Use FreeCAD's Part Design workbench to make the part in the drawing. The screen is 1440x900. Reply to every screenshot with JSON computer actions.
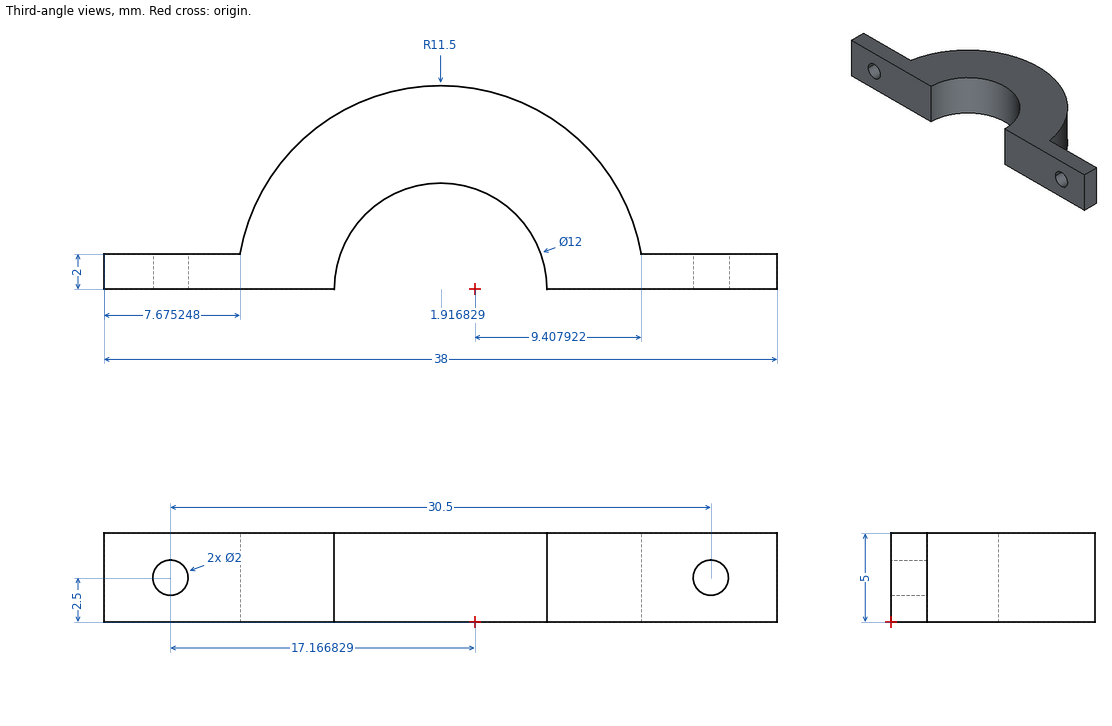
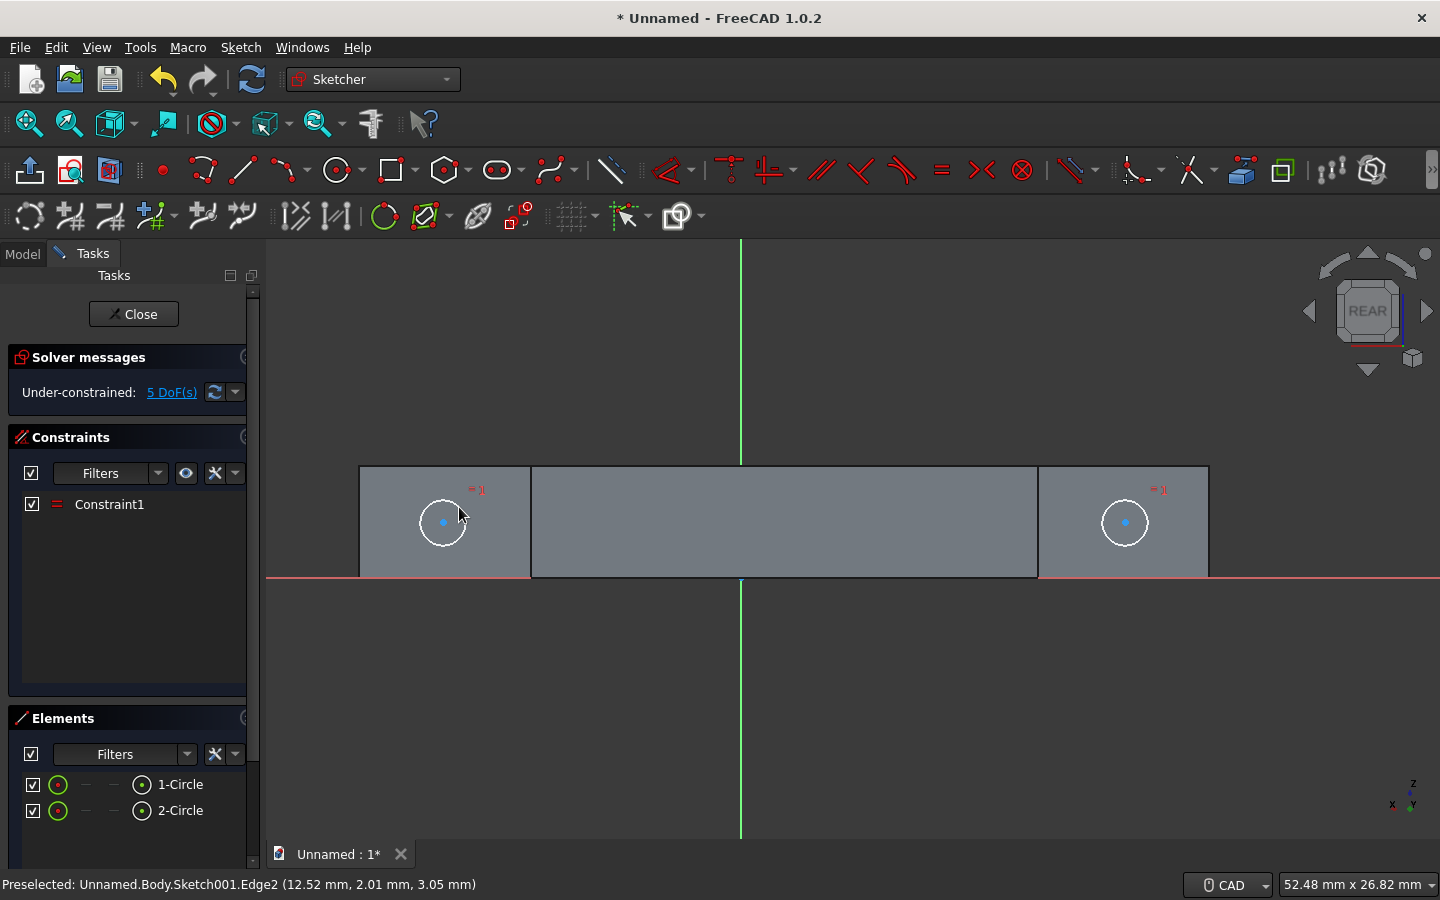
{"action": "left_click", "coordinate": [1125, 523]}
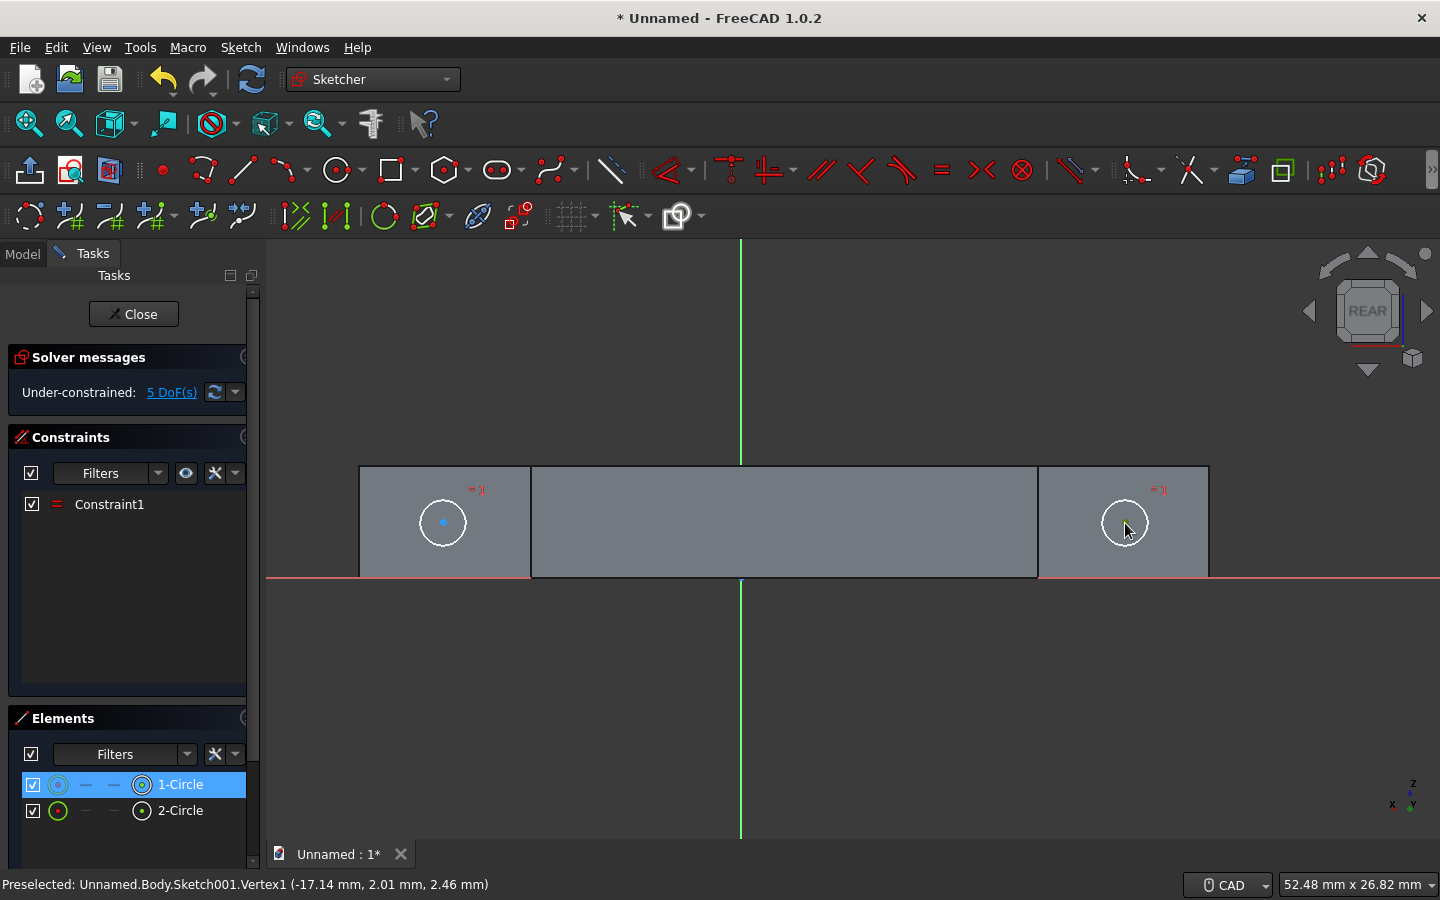
{"action": "left_click", "coordinate": [443, 523]}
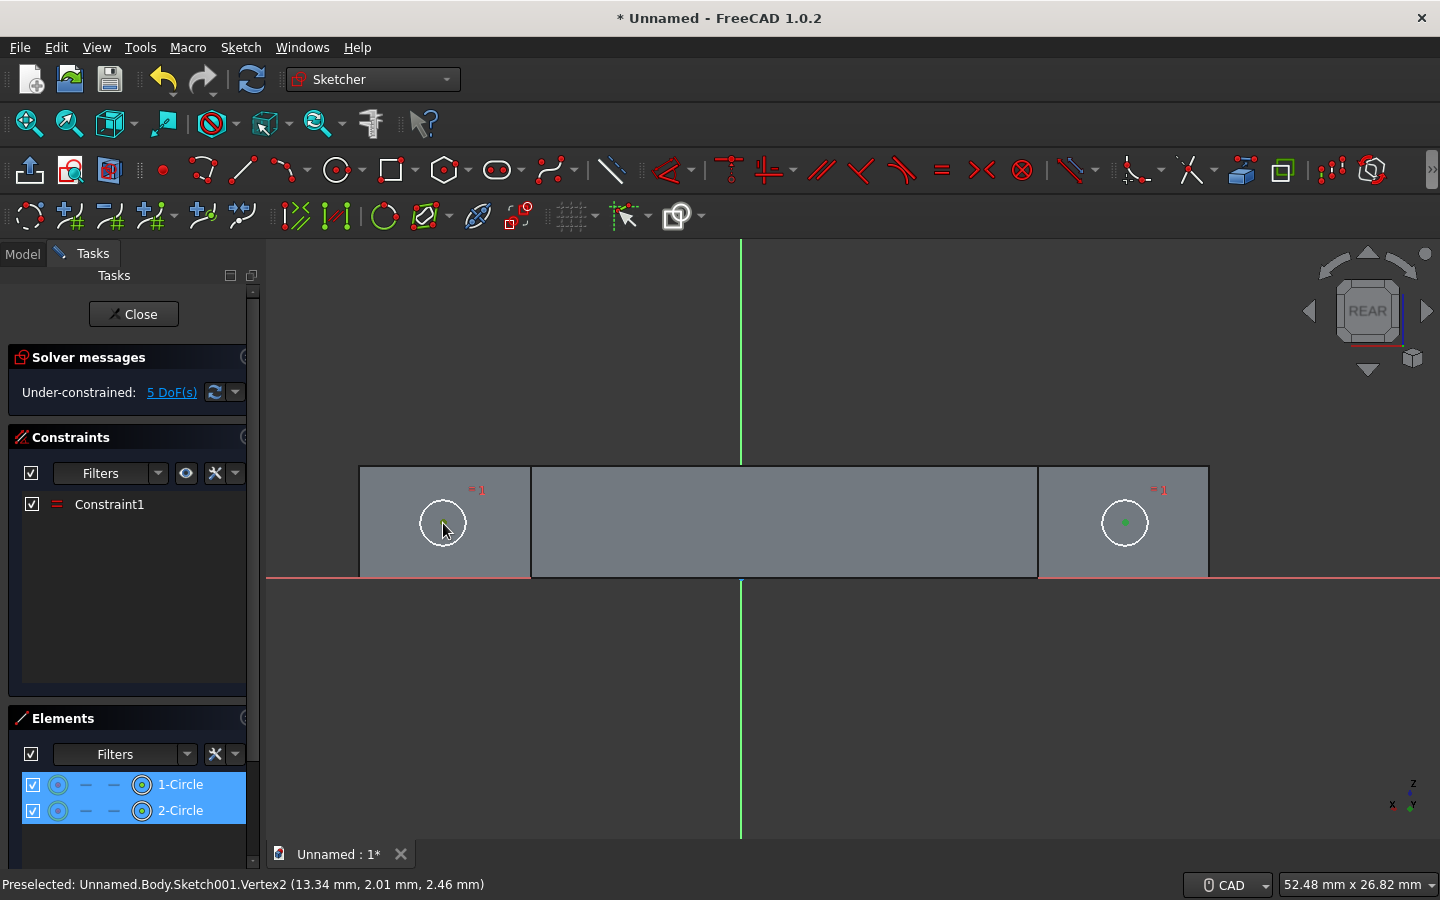
{"action": "key", "text": "h"}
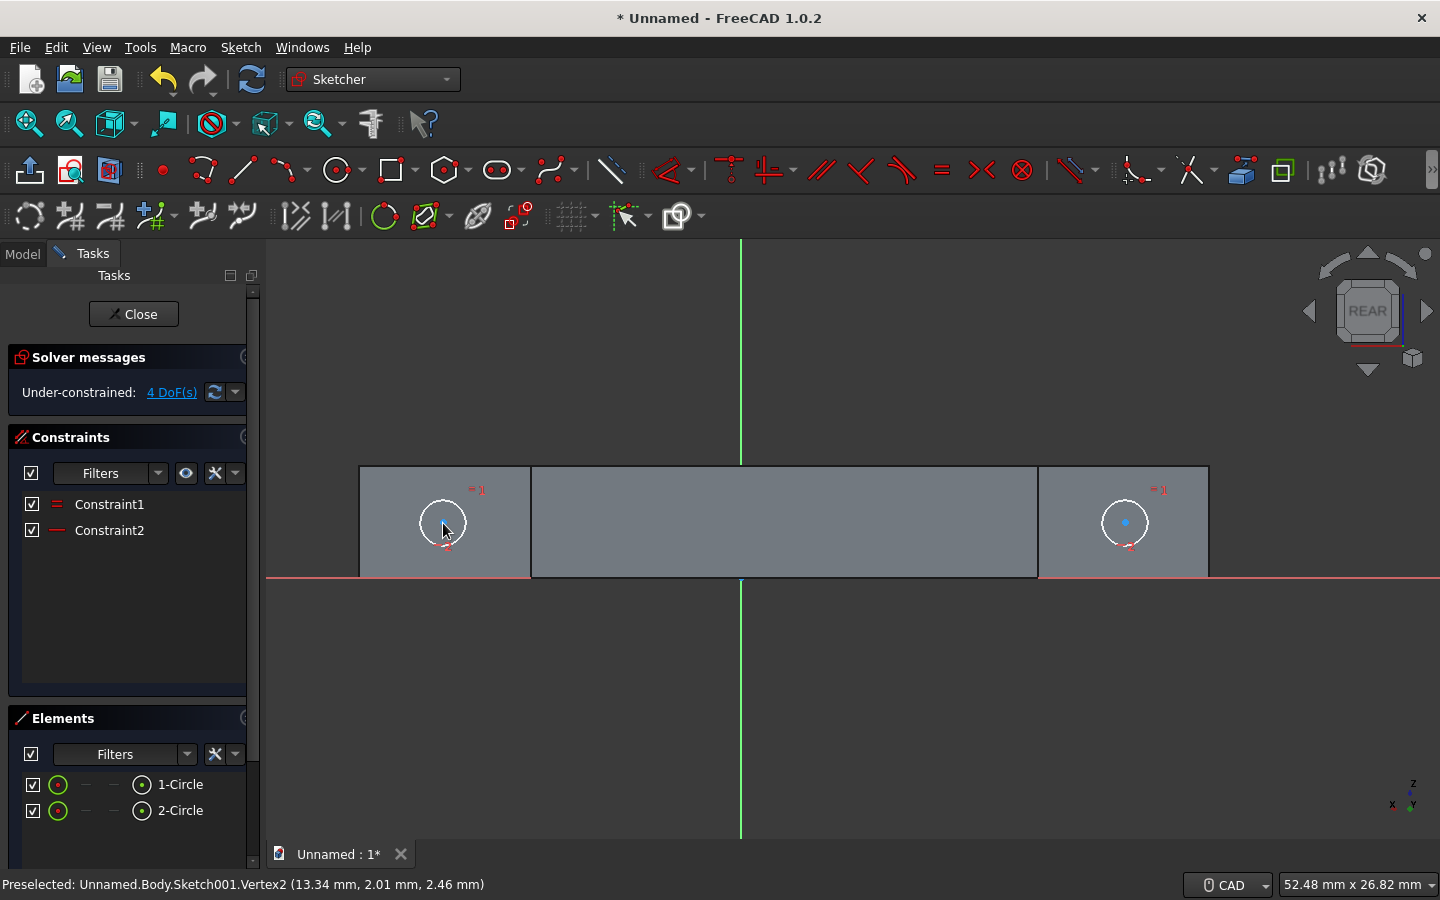
{"action": "left_click", "coordinate": [666, 170]}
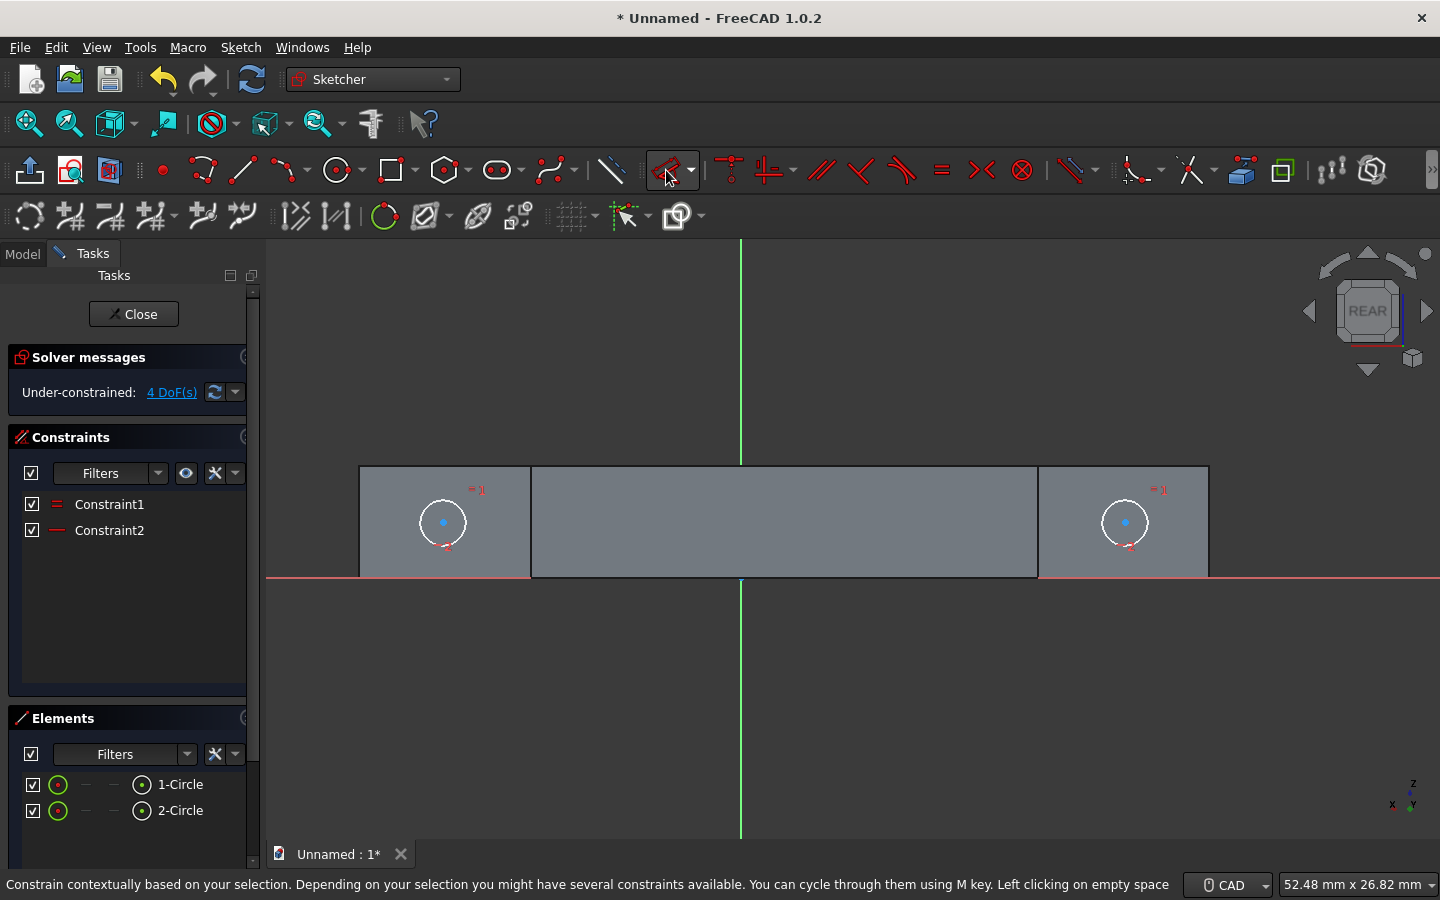
{"action": "left_click", "coordinate": [1141, 507]}
{"action": "left_click", "coordinate": [1164, 484]}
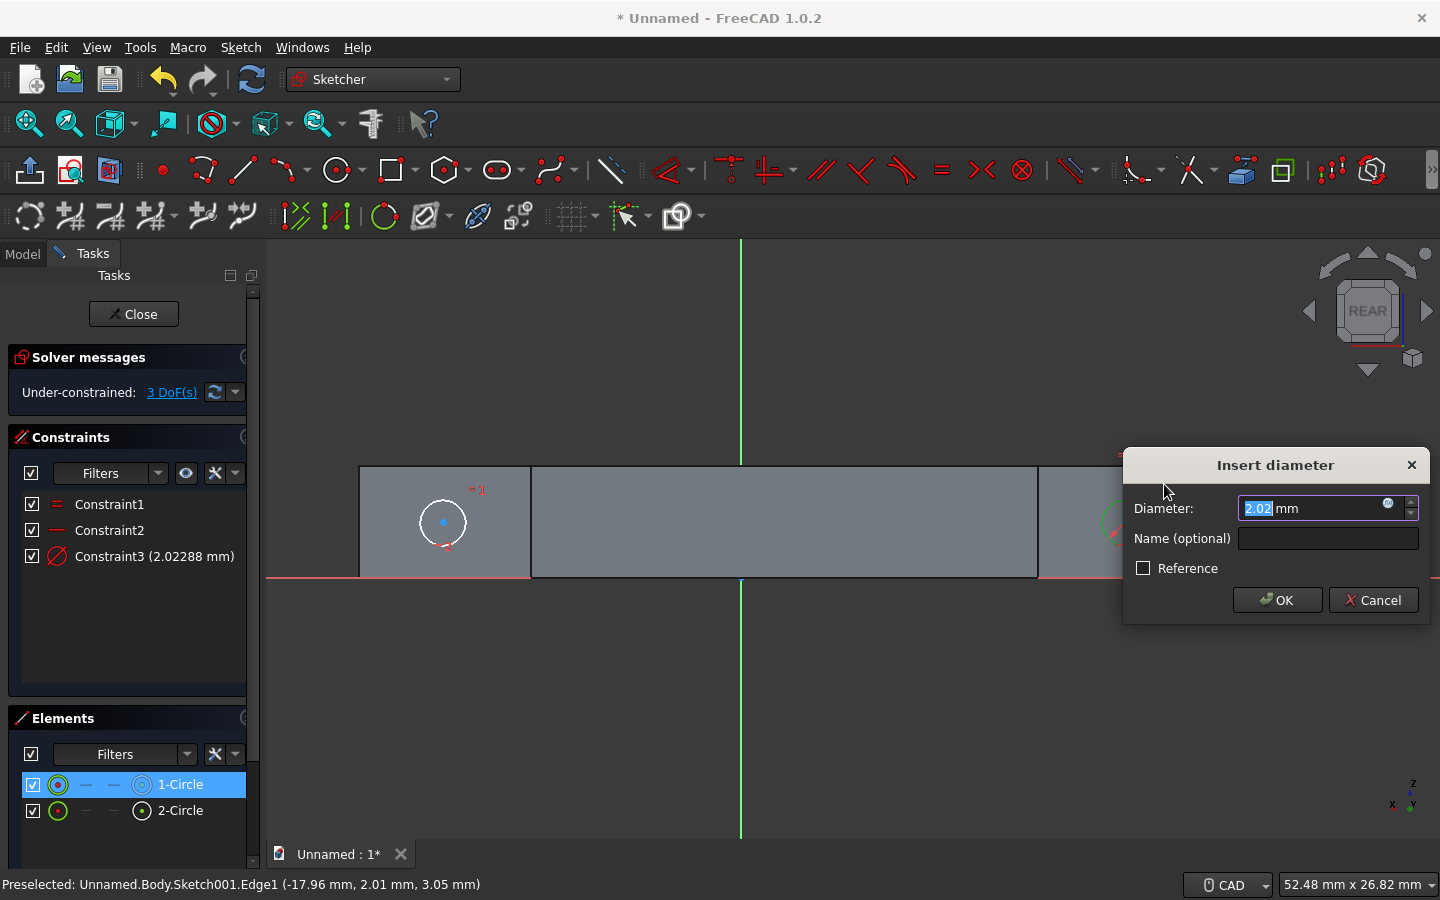
{"action": "type", "text": "2"}
{"action": "key", "text": "Return"}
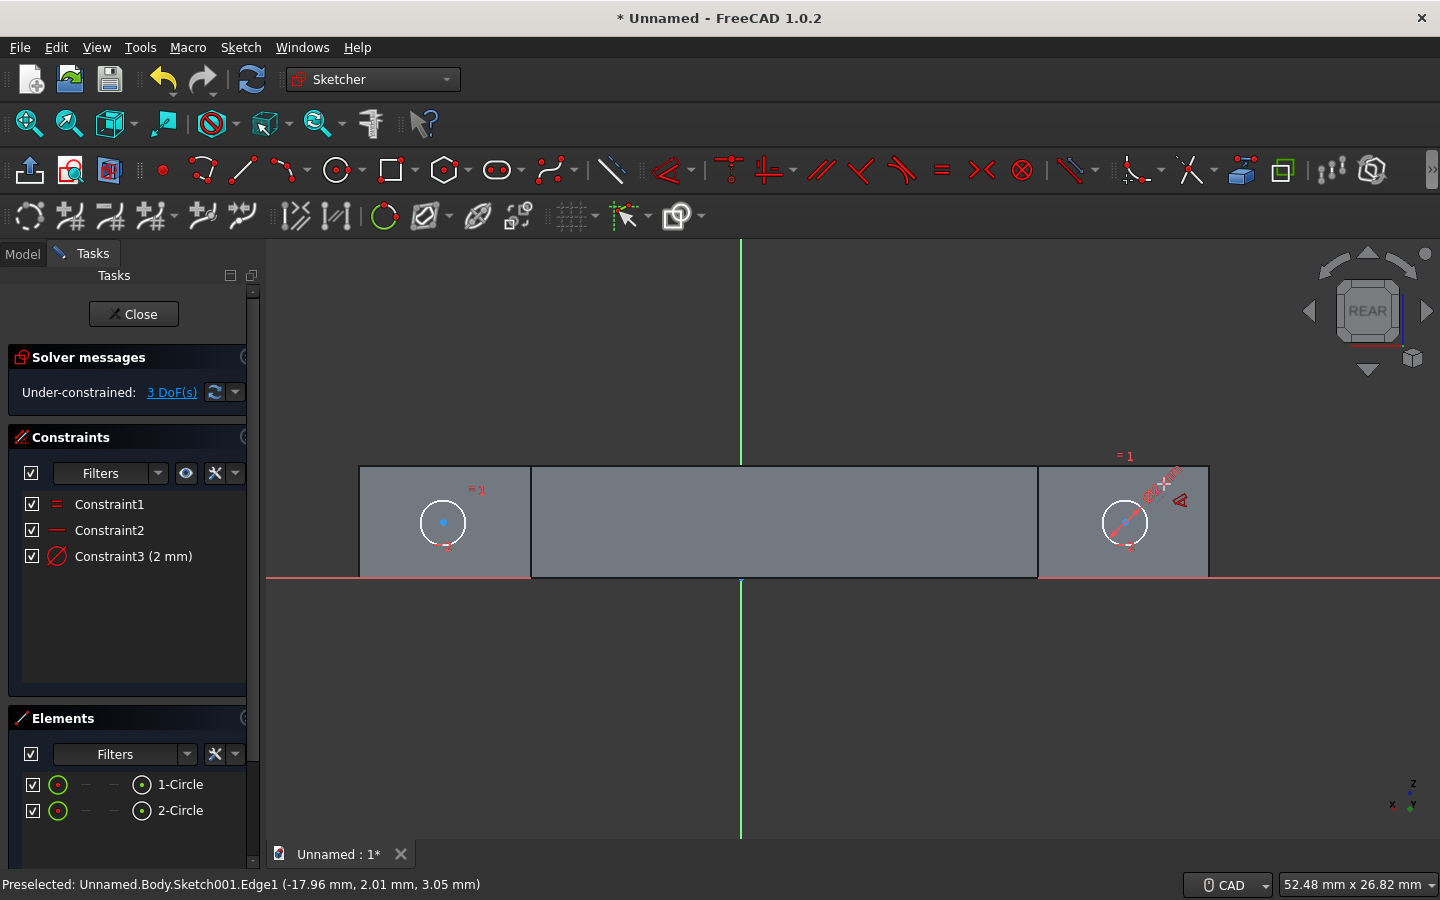
{"action": "left_click", "coordinate": [1125, 523]}
{"action": "left_click", "coordinate": [1159, 550]}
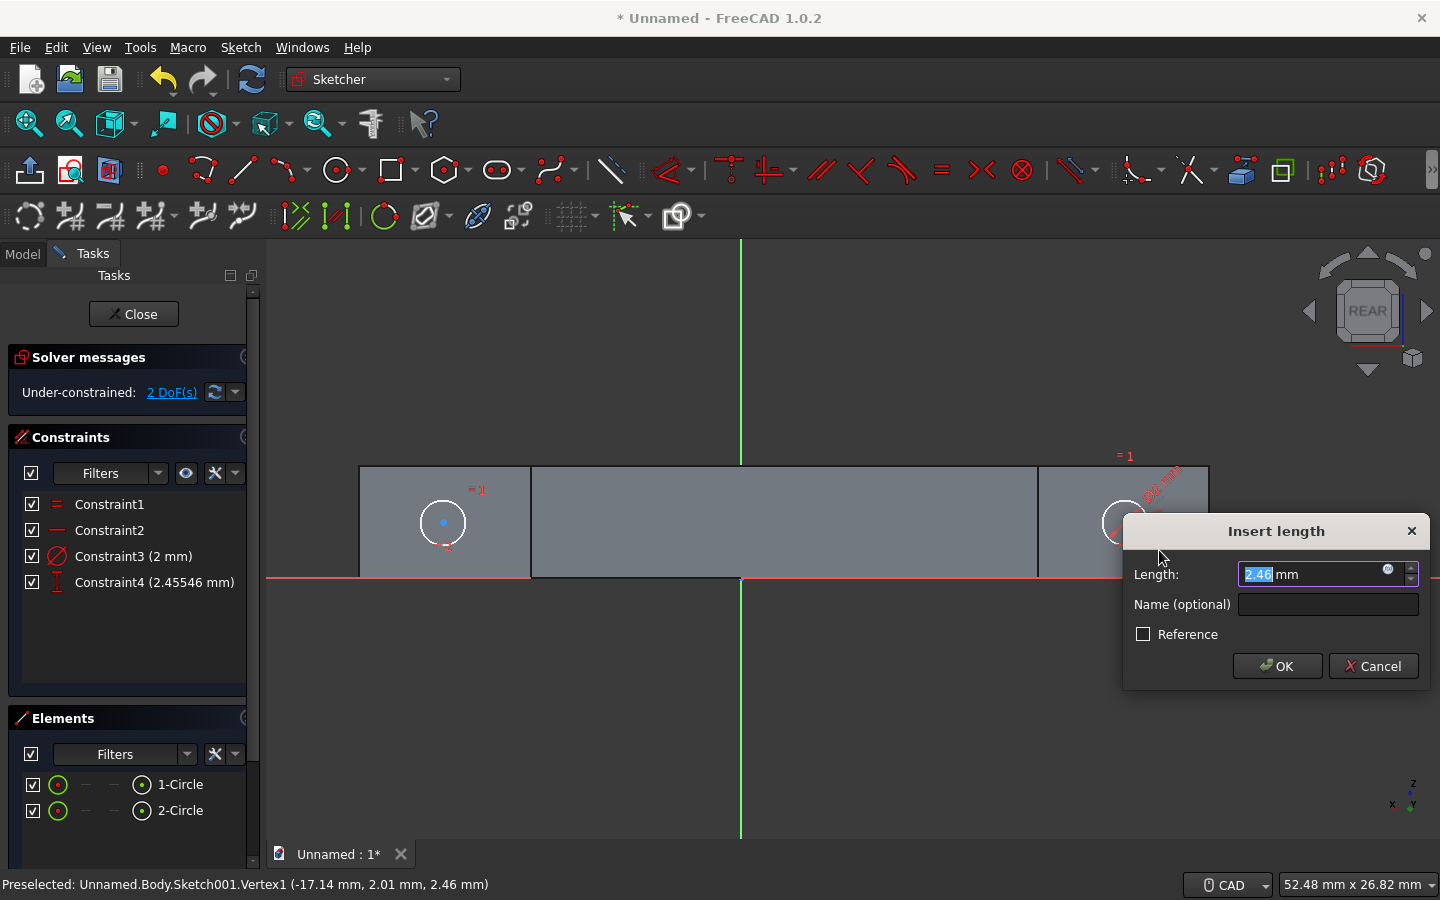
{"action": "type", "text": "2.5"}
{"action": "key", "text": "Return"}